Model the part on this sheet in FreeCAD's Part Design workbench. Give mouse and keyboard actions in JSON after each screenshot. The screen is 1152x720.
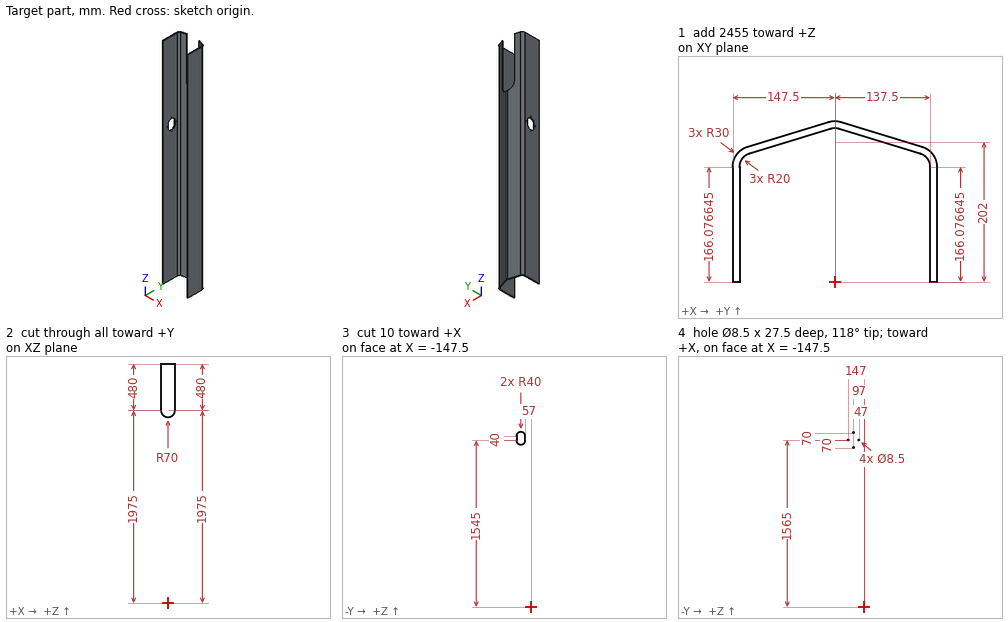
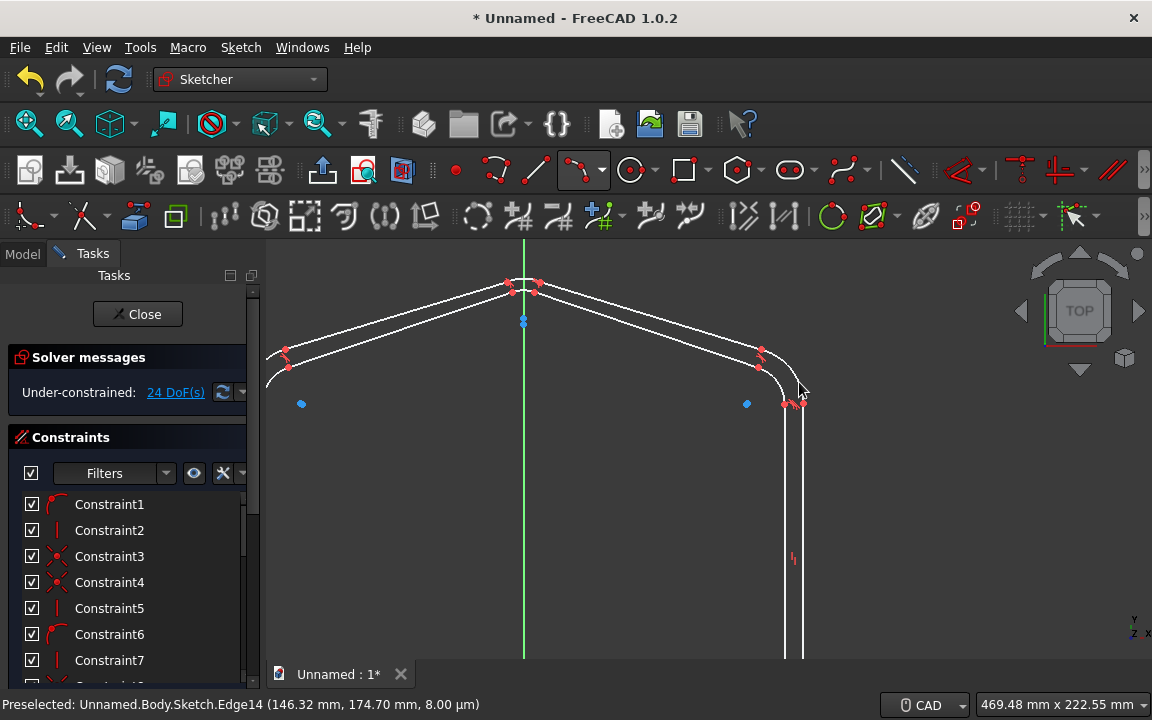
{"action": "left_click", "coordinate": [696, 330]}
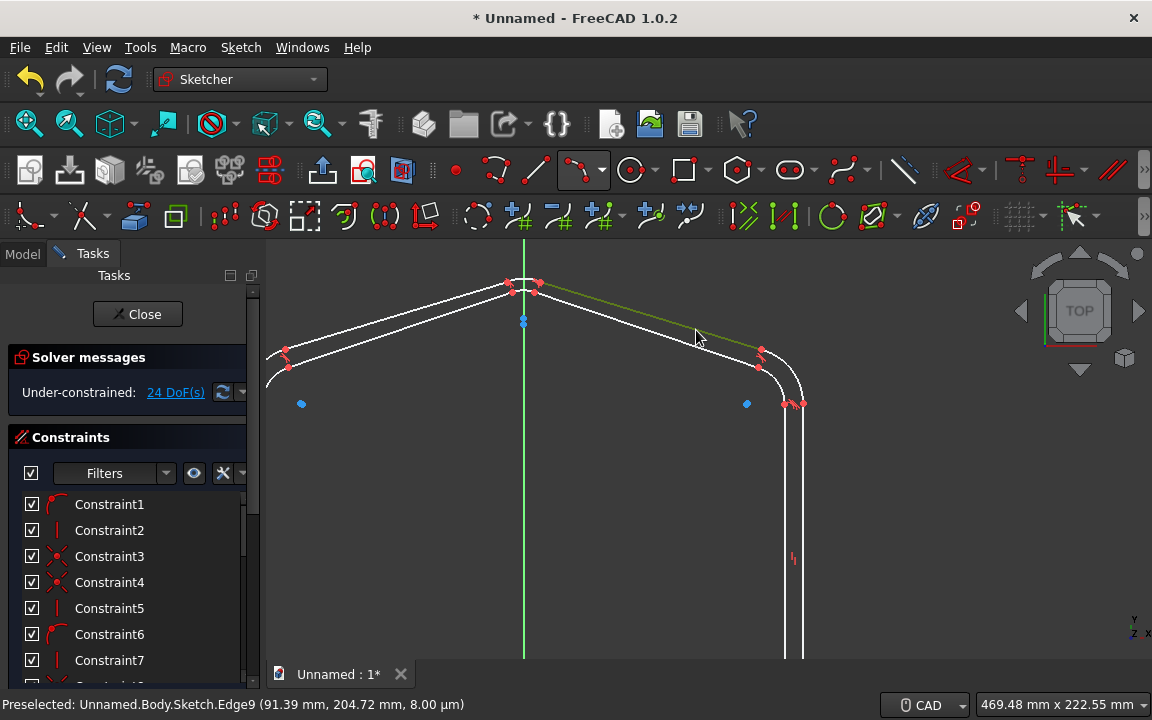
{"action": "left_click", "coordinate": [799, 382]}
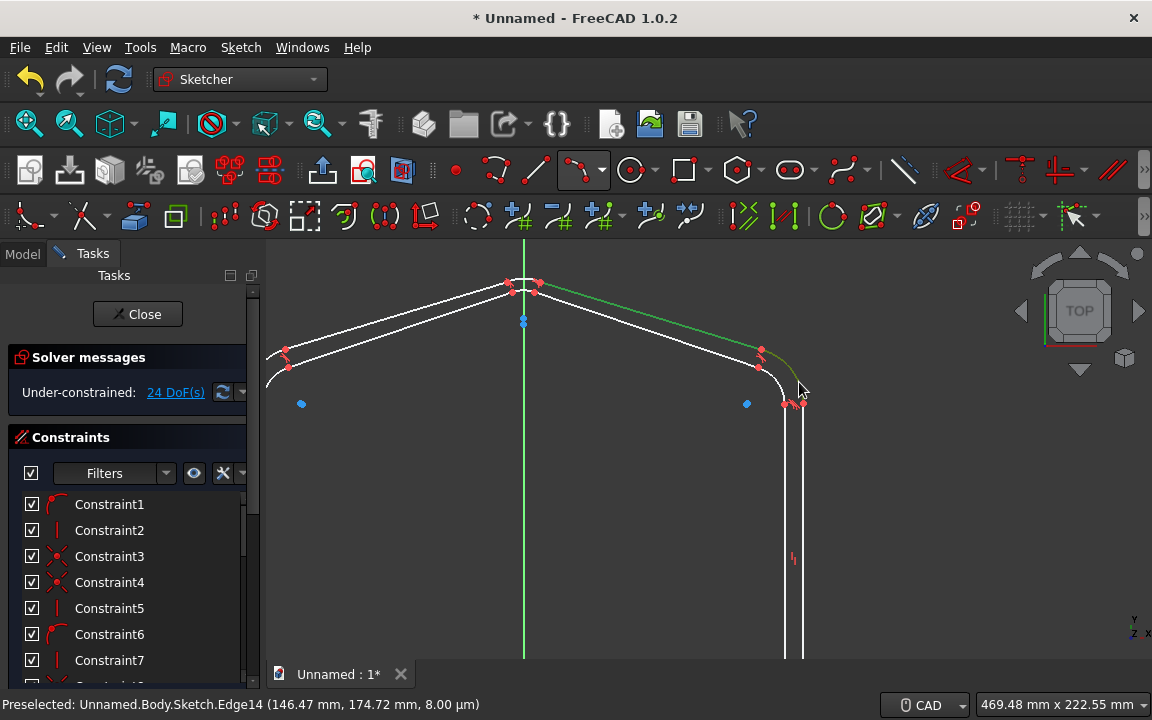
{"action": "key", "text": "t"}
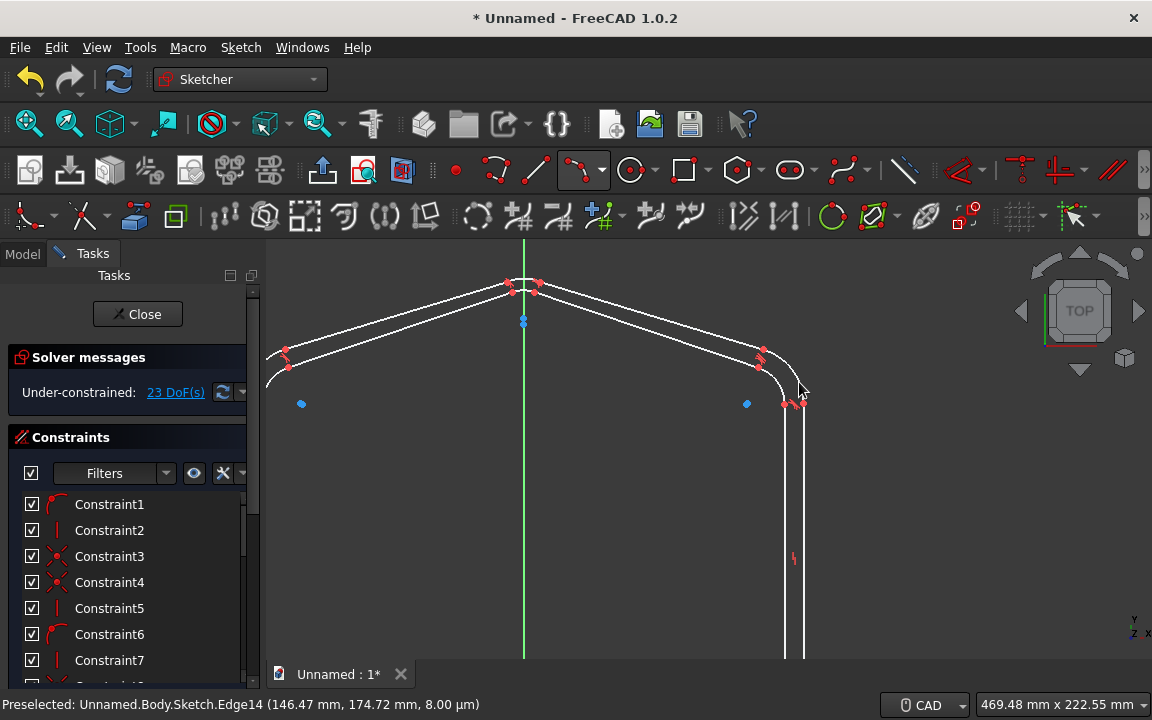
{"action": "left_click", "coordinate": [697, 330]}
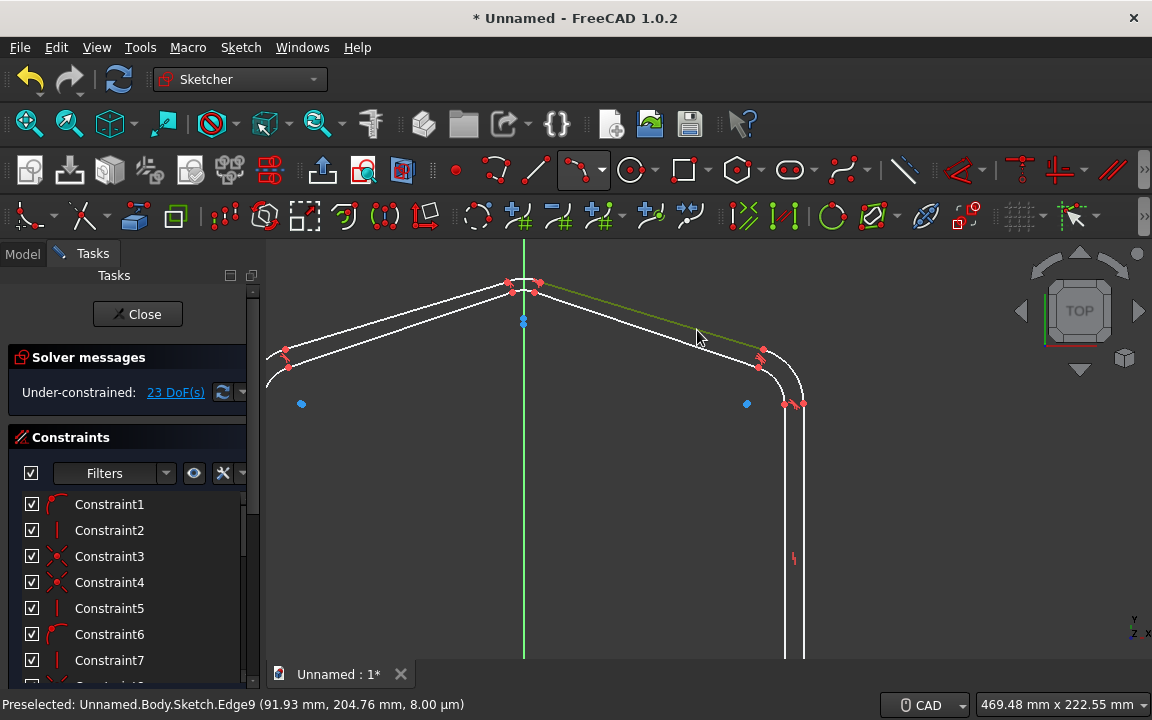
{"action": "left_click", "coordinate": [524, 279]}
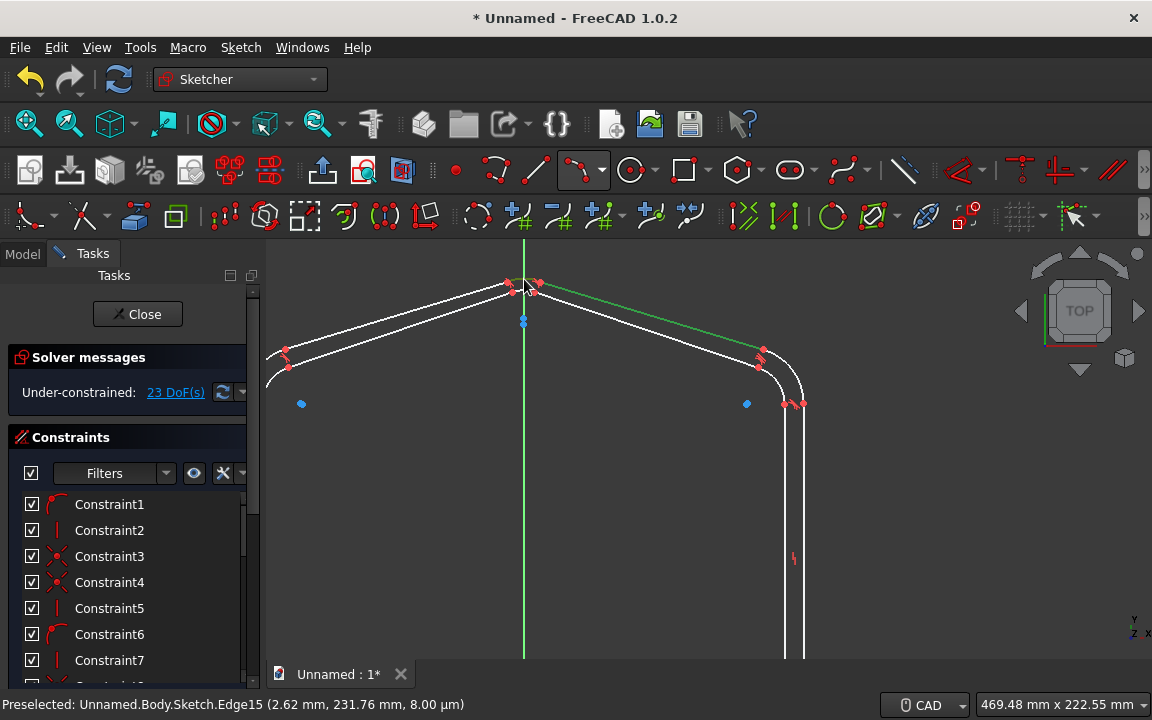
{"action": "key", "text": "t"}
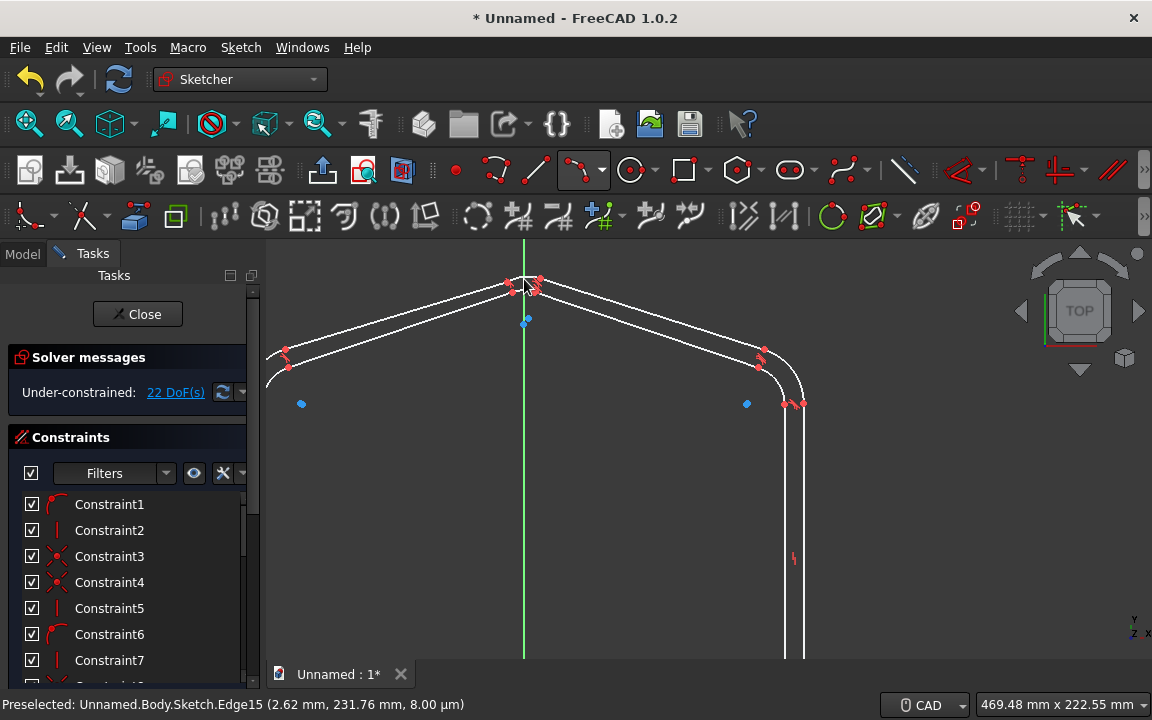
{"action": "left_click", "coordinate": [441, 302]}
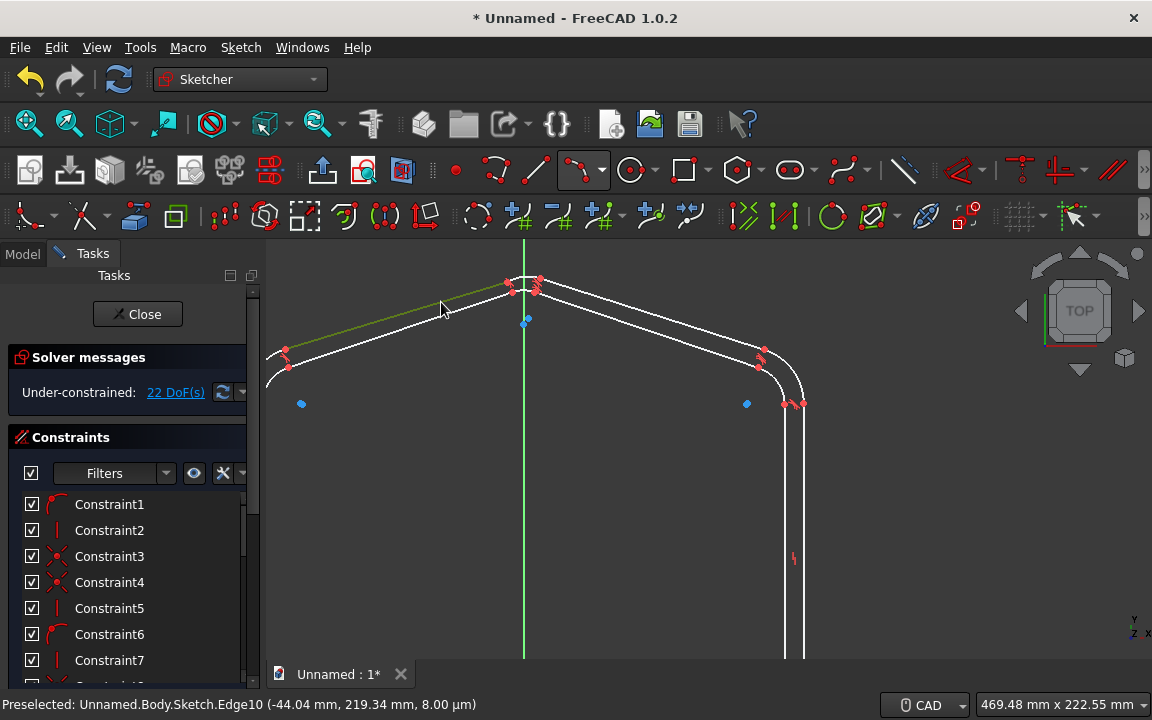
{"action": "left_click", "coordinate": [524, 277]}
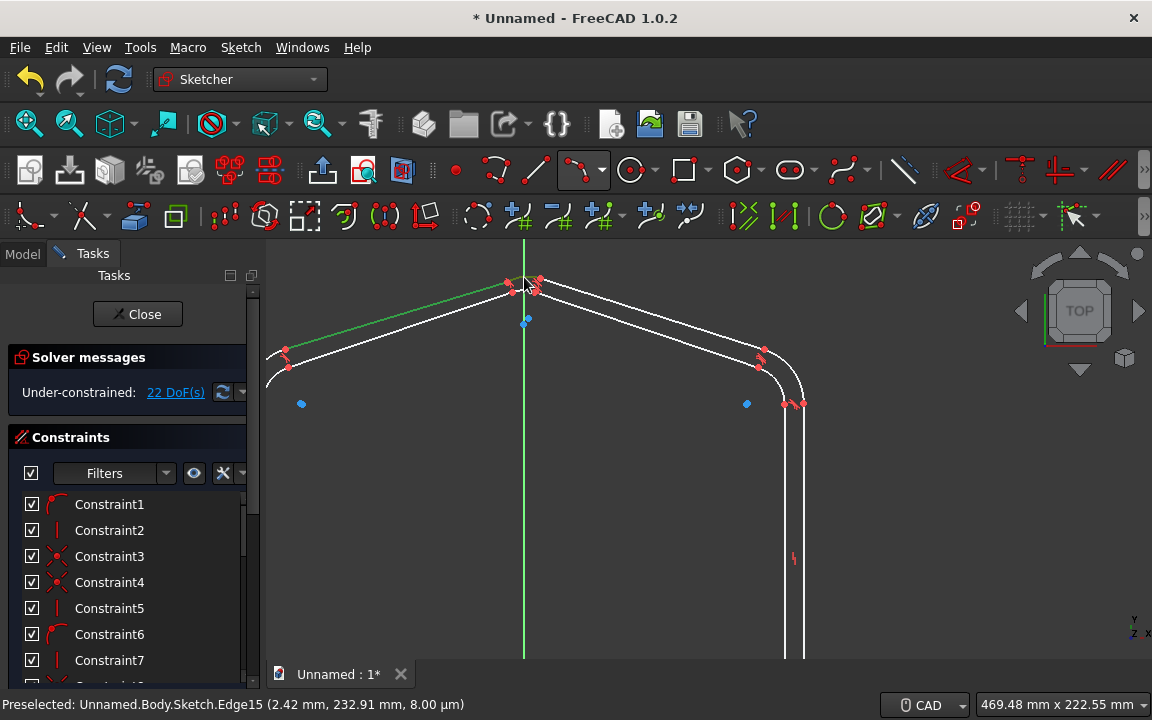
{"action": "key", "text": "t"}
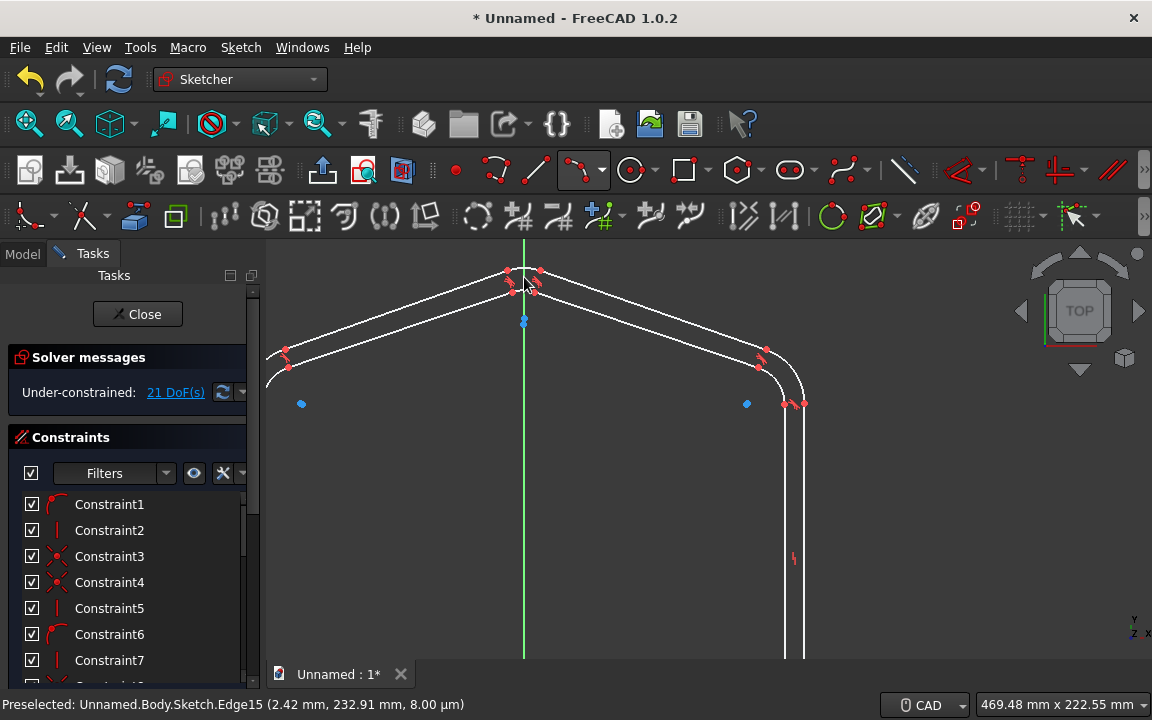
{"action": "left_click", "coordinate": [441, 294]}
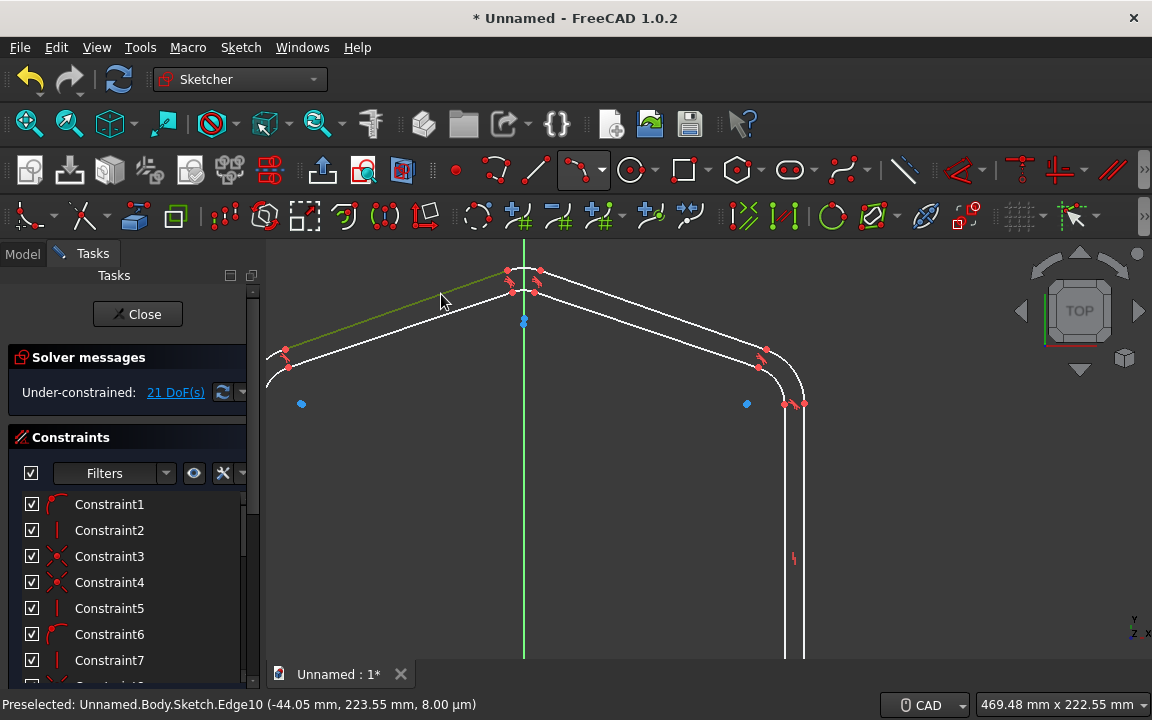
{"action": "scroll", "coordinate": [782, 390], "scroll_direction": "down", "scroll_amount": 3}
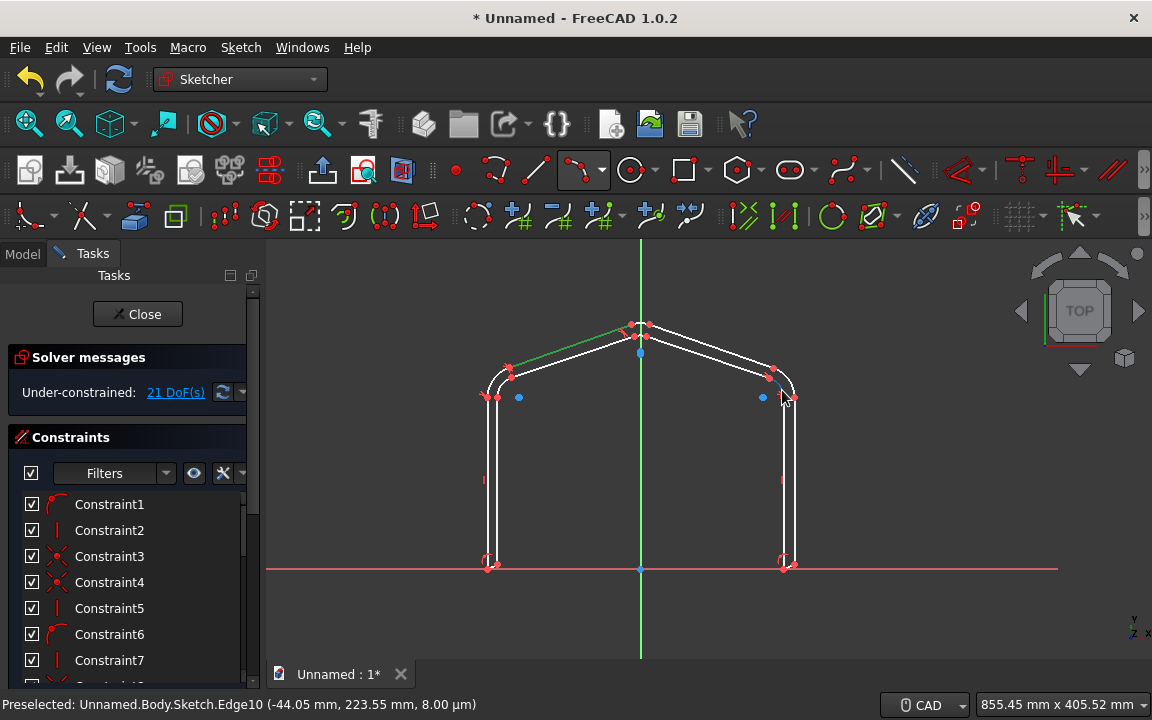
{"action": "scroll", "coordinate": [499, 373], "scroll_direction": "up", "scroll_amount": 2}